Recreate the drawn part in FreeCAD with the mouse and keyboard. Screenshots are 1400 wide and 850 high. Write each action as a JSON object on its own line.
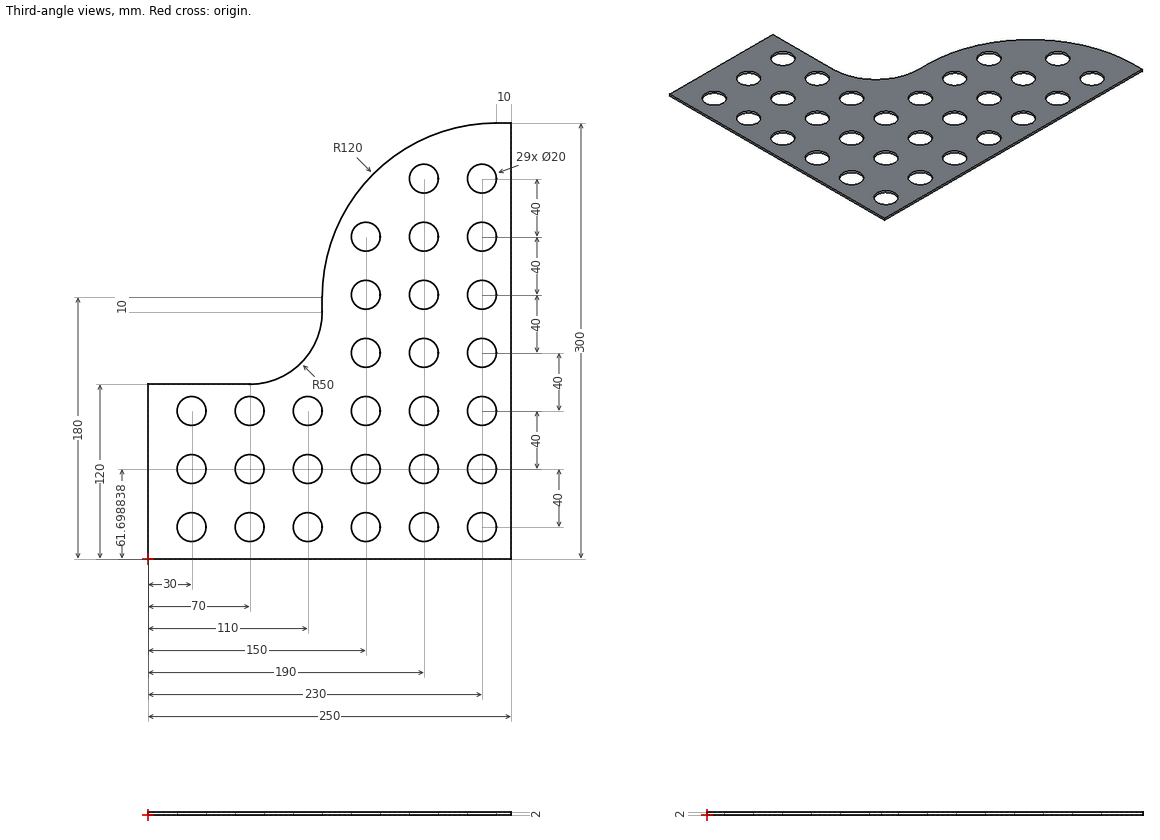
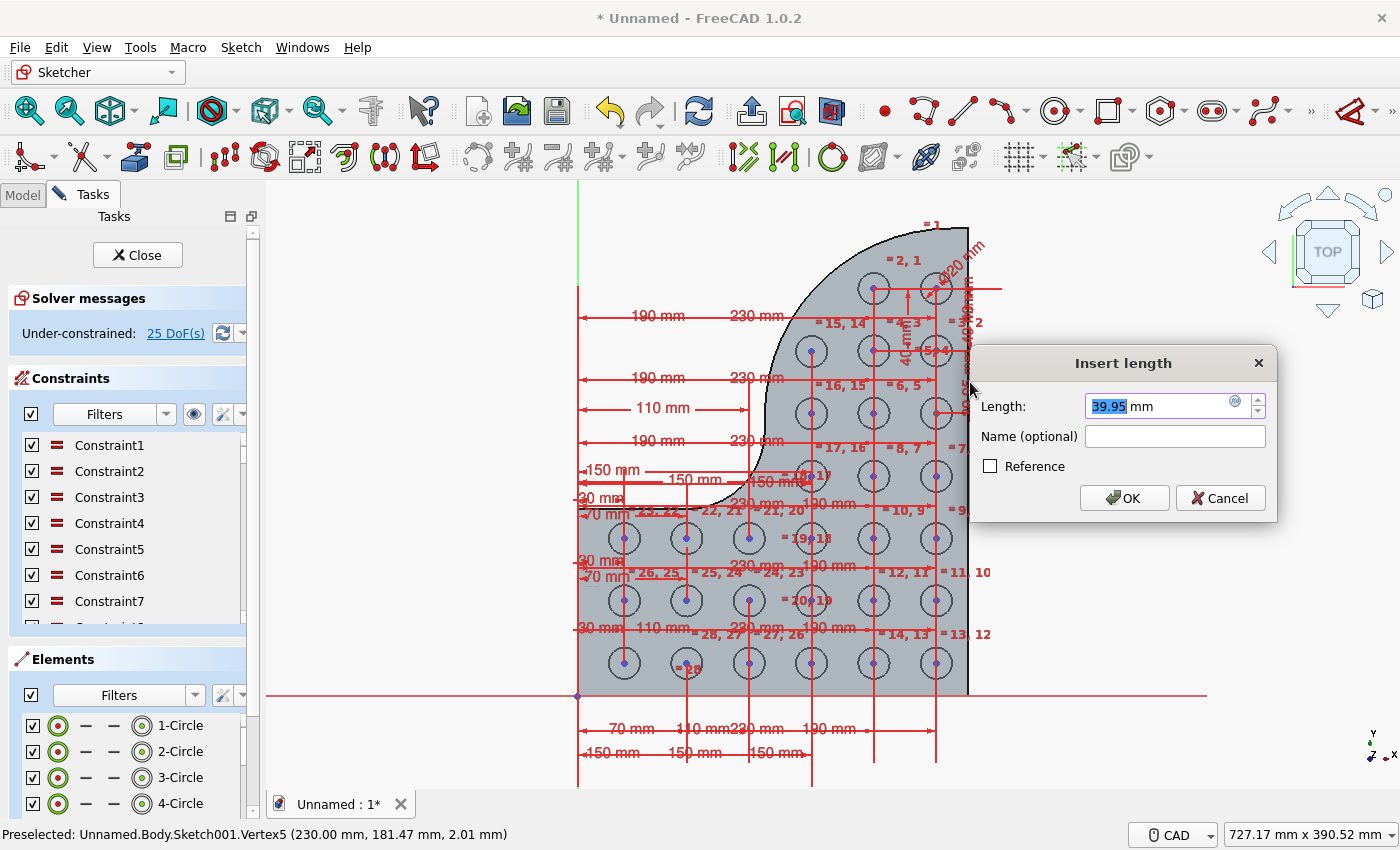
{"action": "type", "text": "40"}
{"action": "key", "text": "Return"}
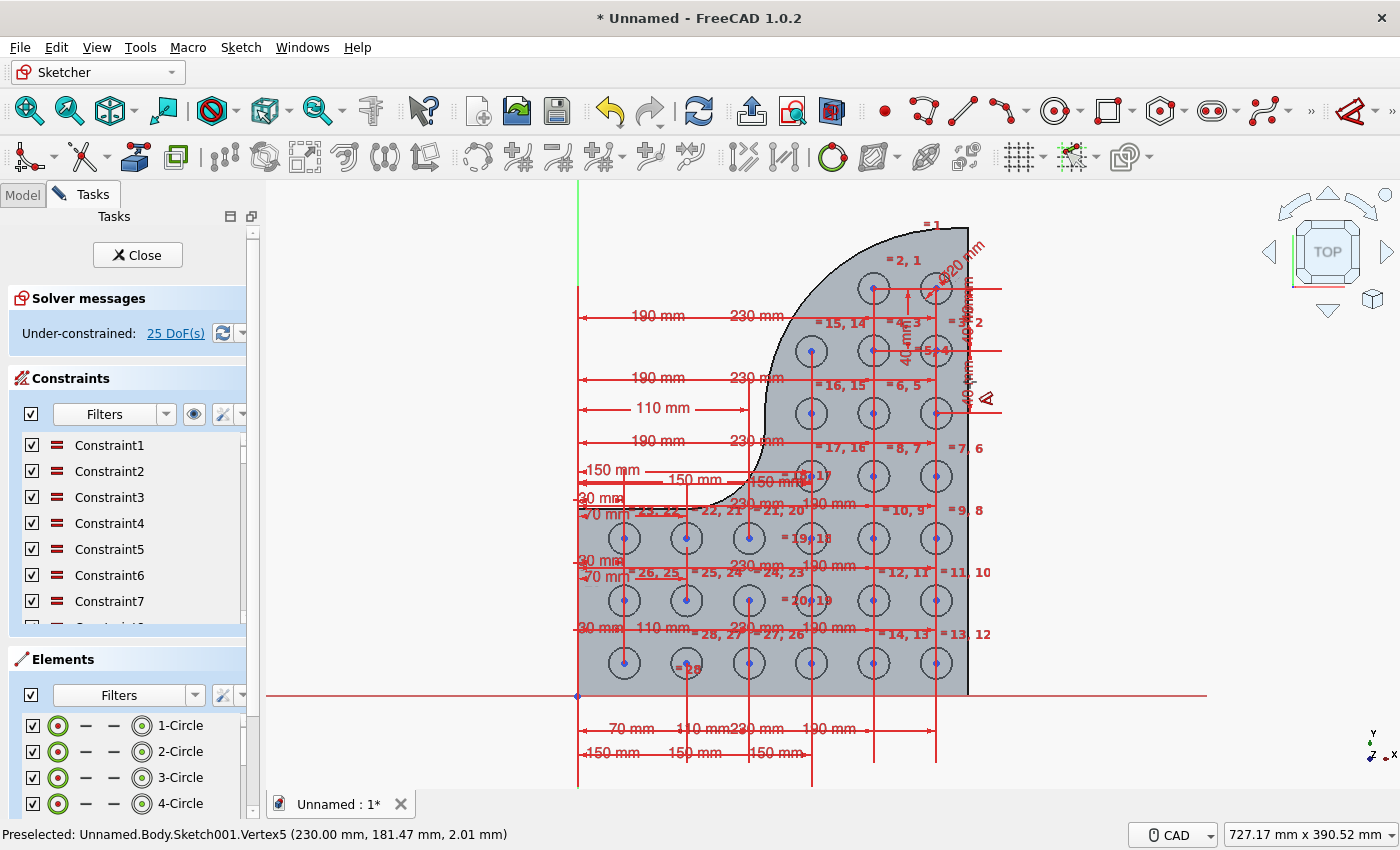
{"action": "left_click", "coordinate": [874, 351]}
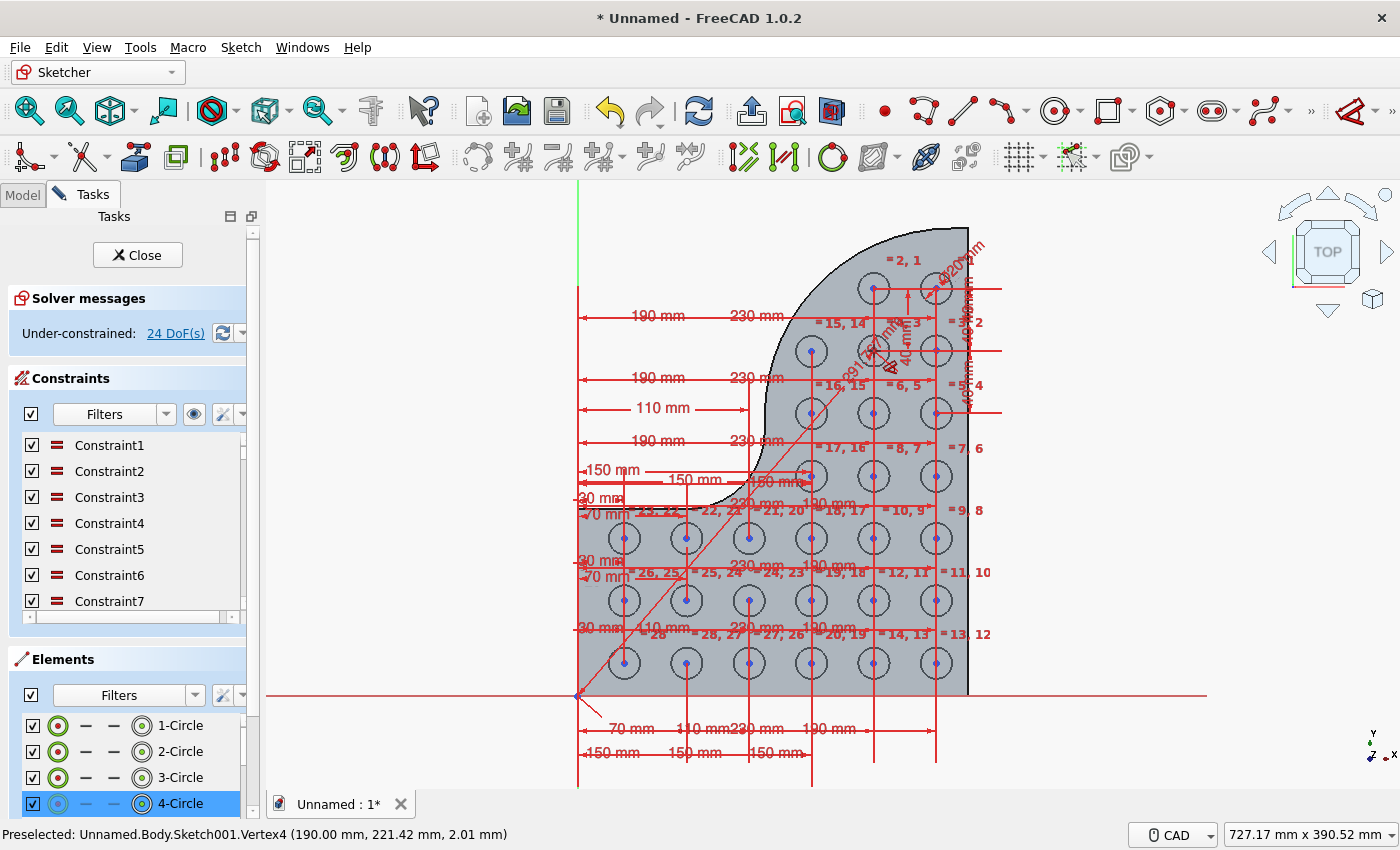
{"action": "left_click", "coordinate": [874, 413]}
{"action": "left_click", "coordinate": [908, 404]}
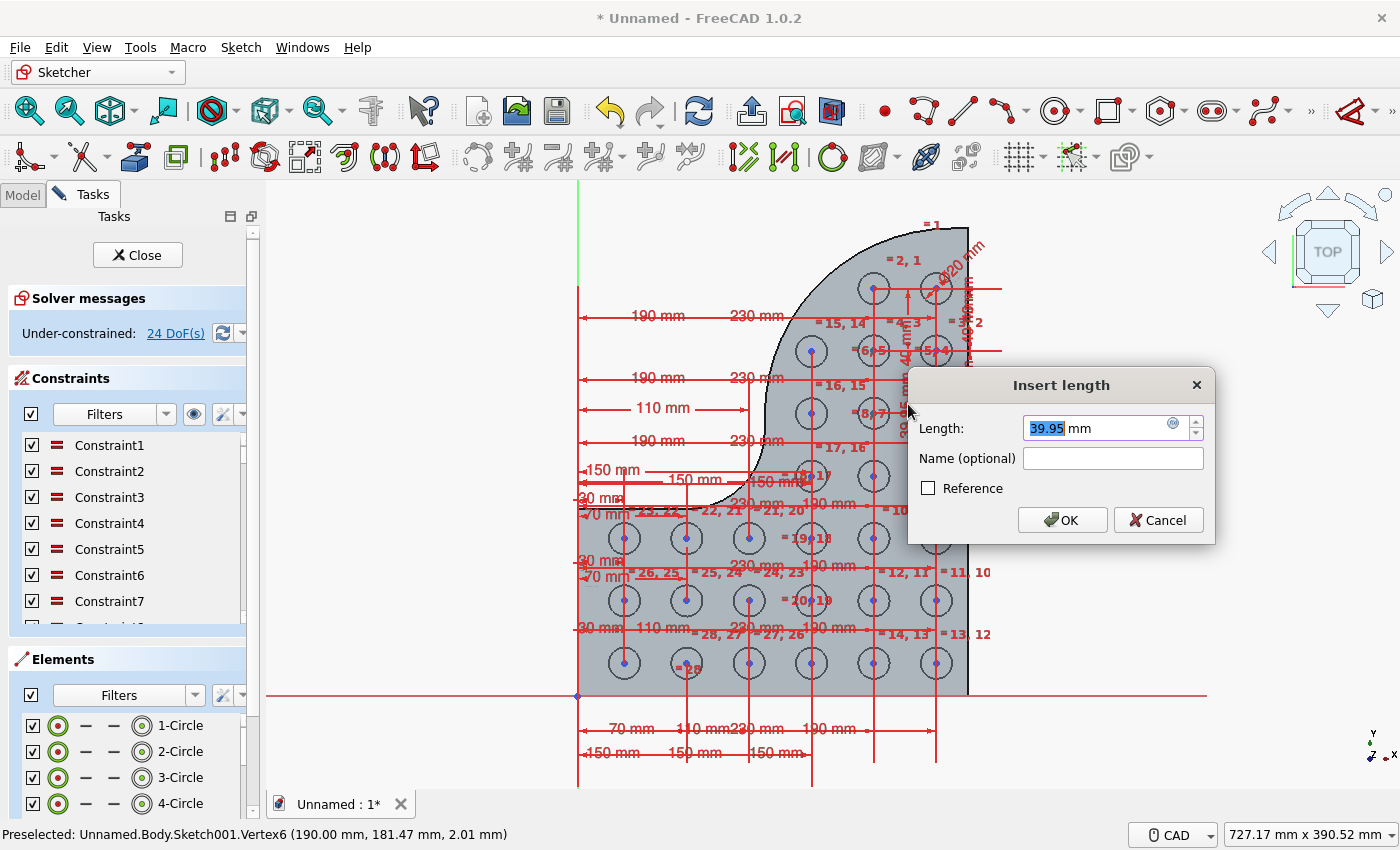
{"action": "type", "text": "40"}
{"action": "key", "text": "Return"}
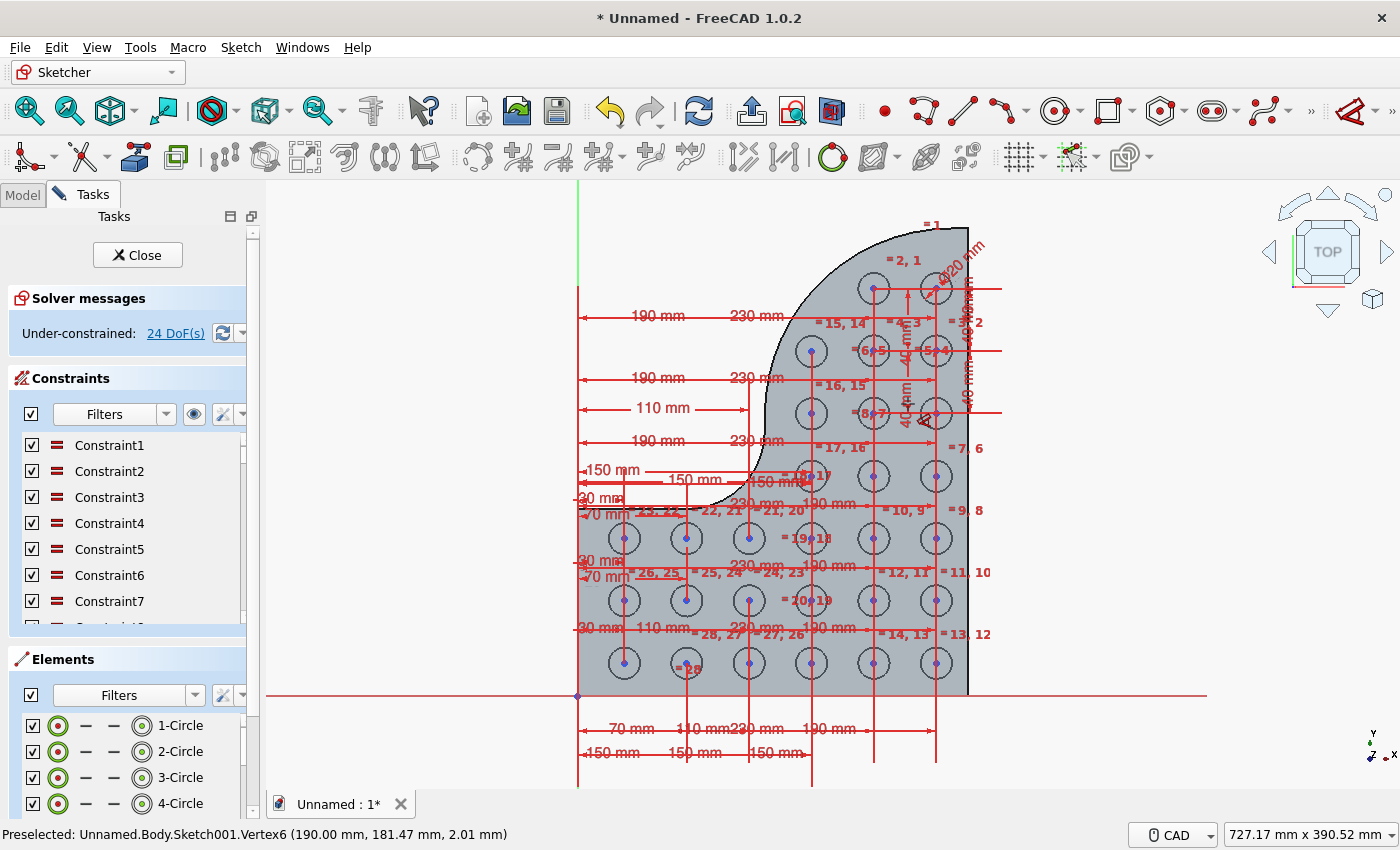
{"action": "left_click", "coordinate": [936, 413]}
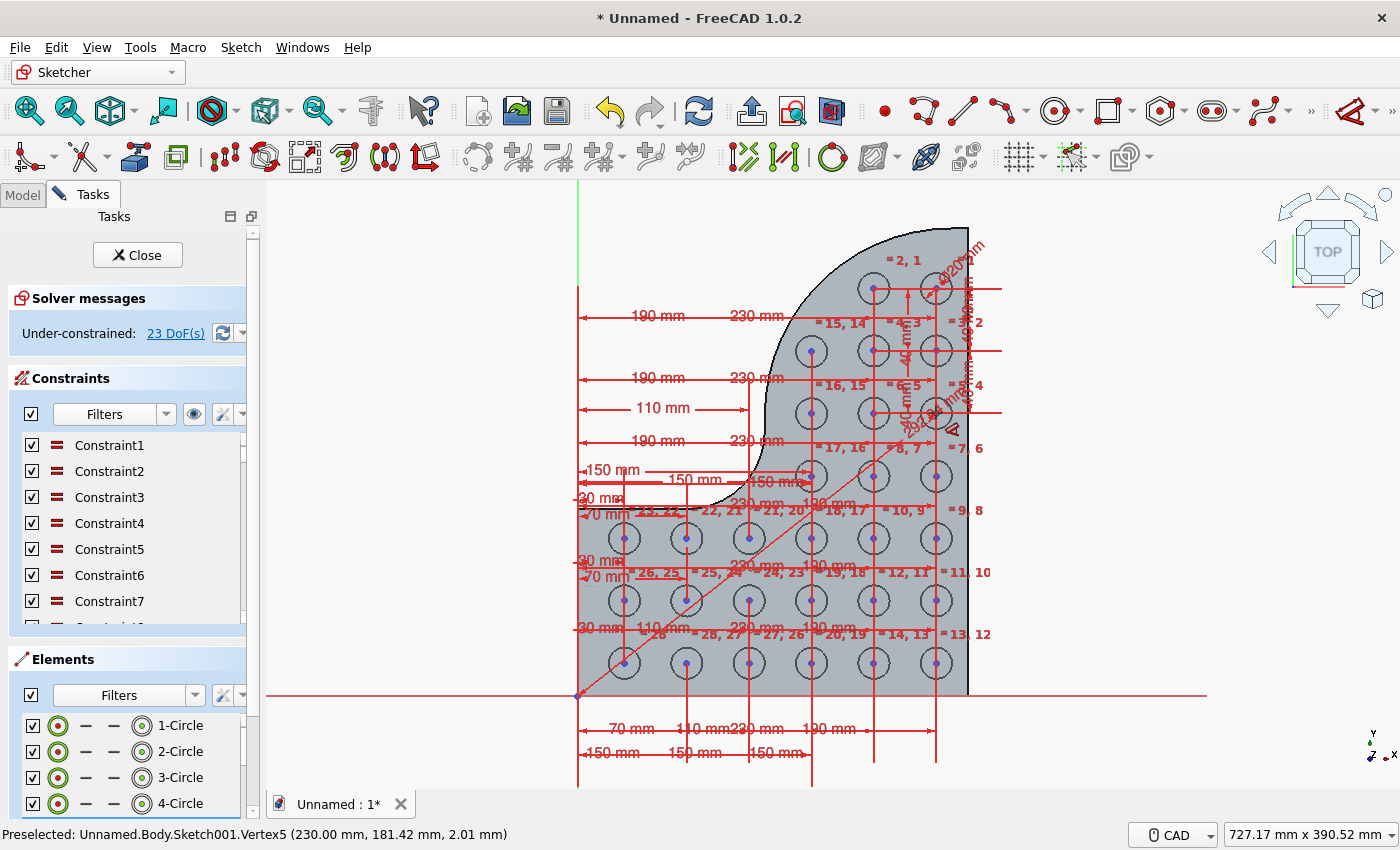
{"action": "left_click", "coordinate": [936, 476]}
{"action": "left_click", "coordinate": [970, 445]}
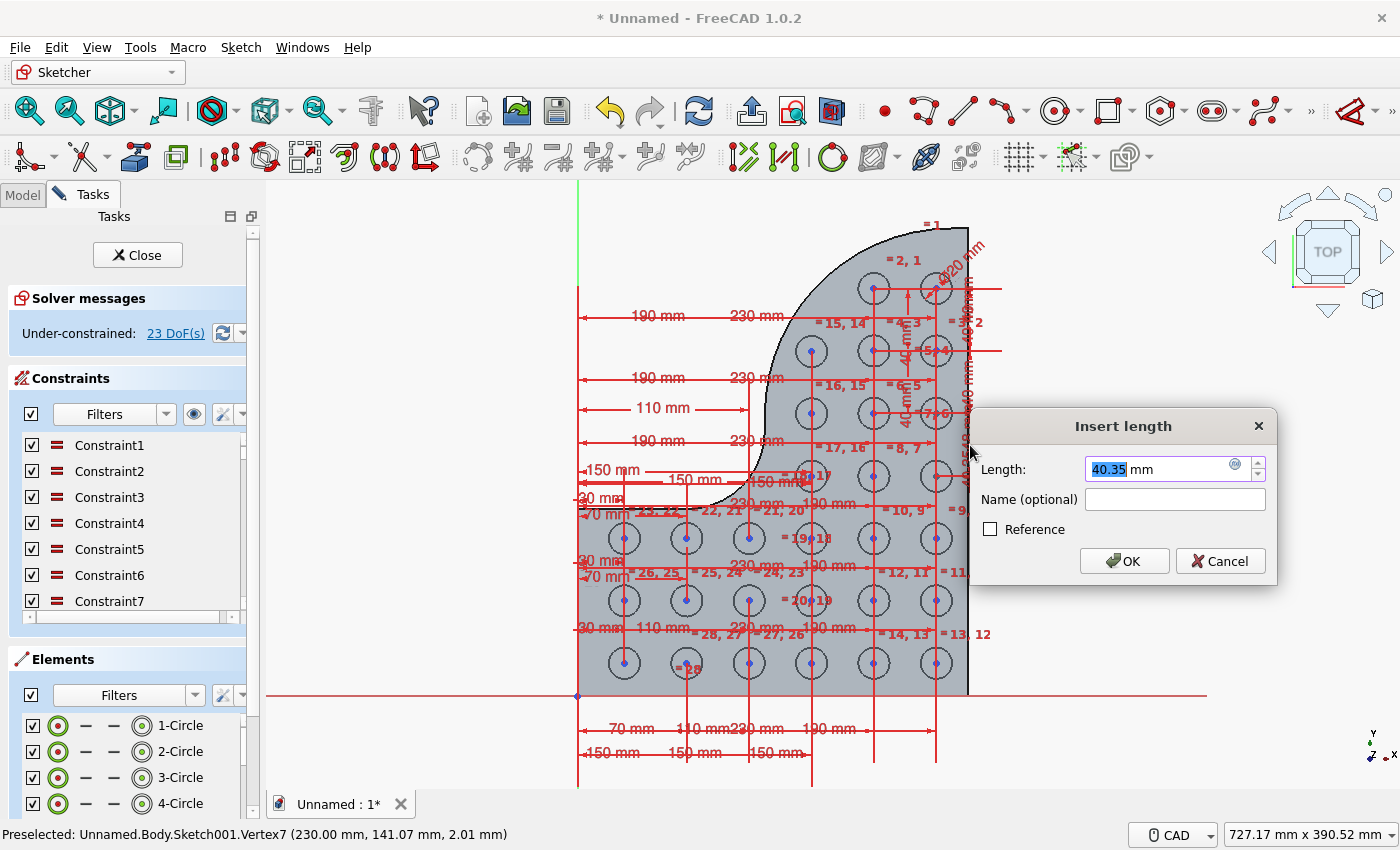
{"action": "type", "text": "40"}
{"action": "key", "text": "Return"}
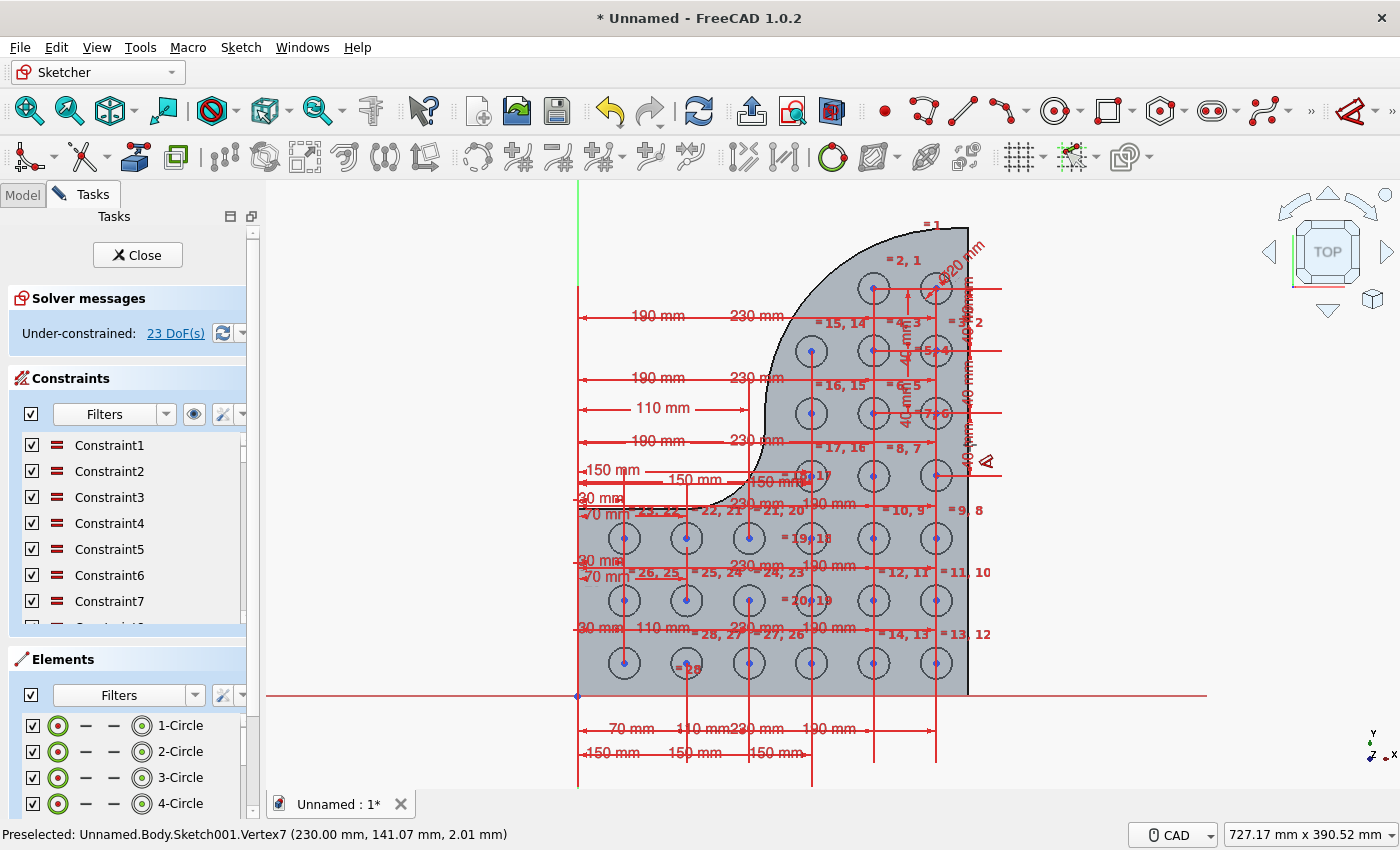
{"action": "left_click", "coordinate": [874, 413]}